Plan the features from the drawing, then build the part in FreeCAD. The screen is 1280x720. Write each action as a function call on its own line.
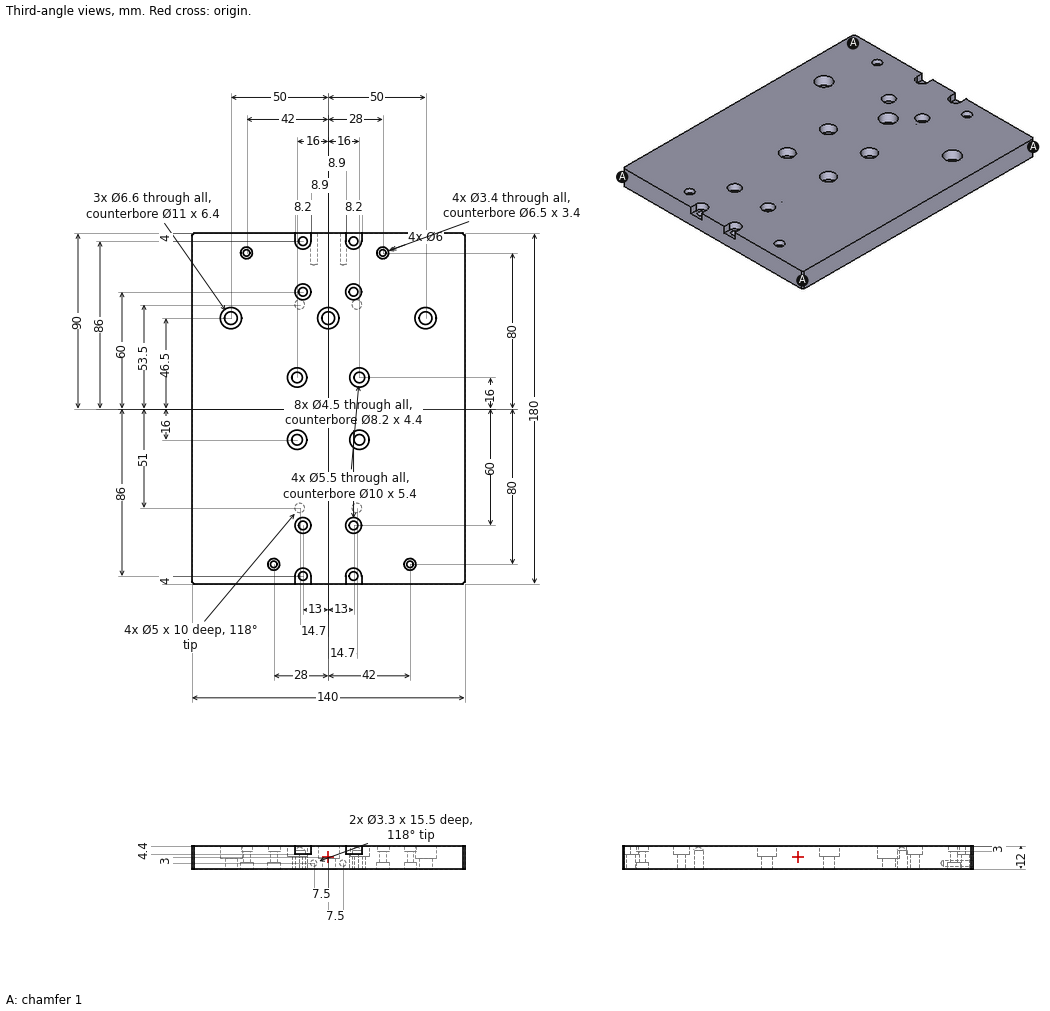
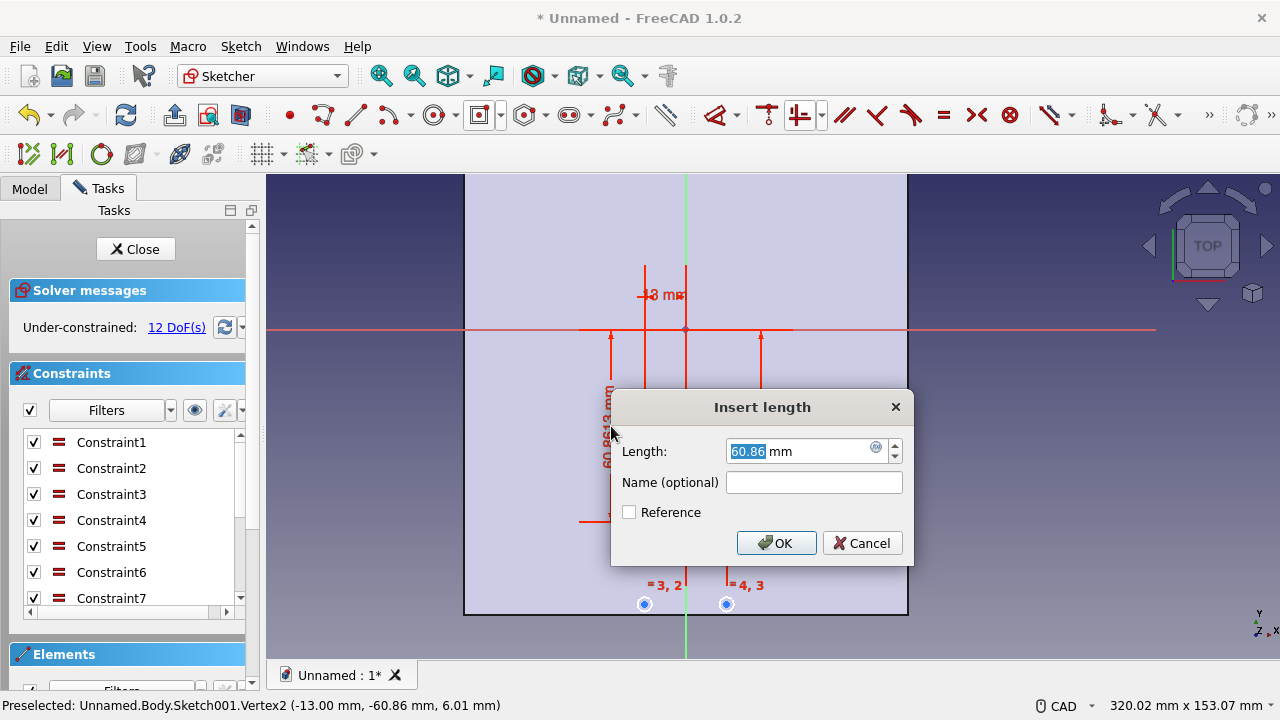
text(60)
key(Return)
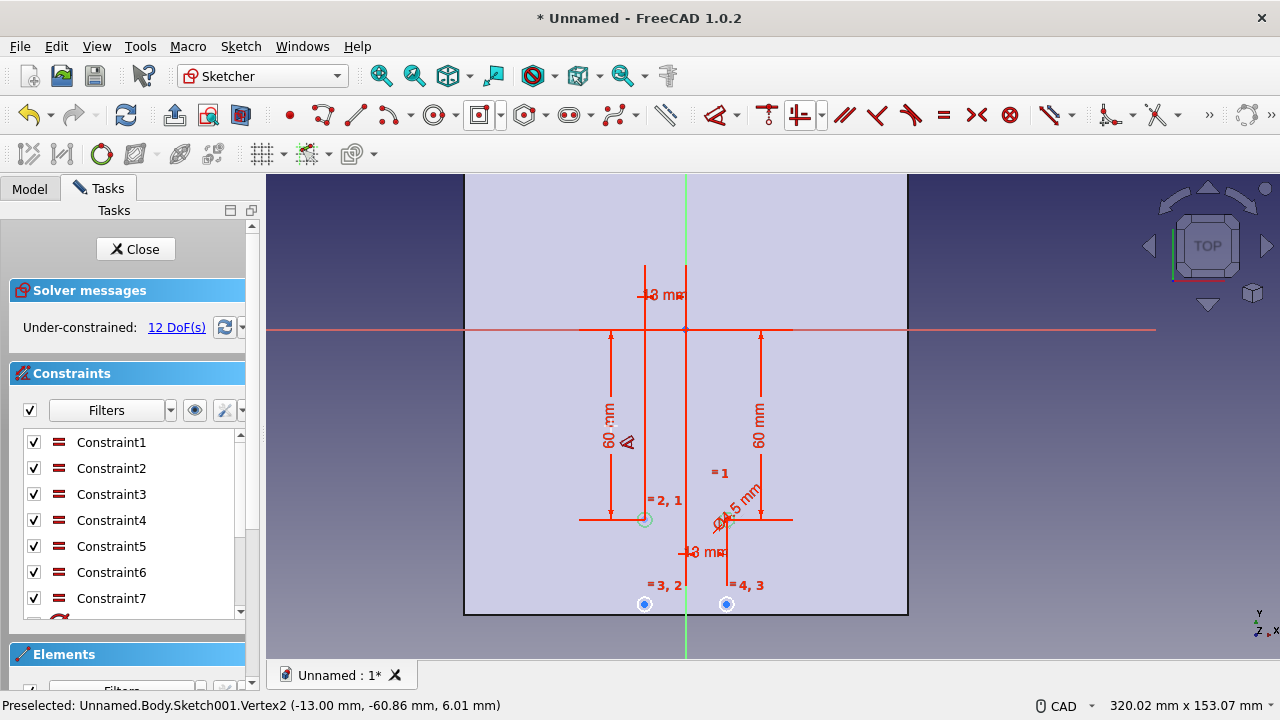
click(645, 604)
click(665, 272)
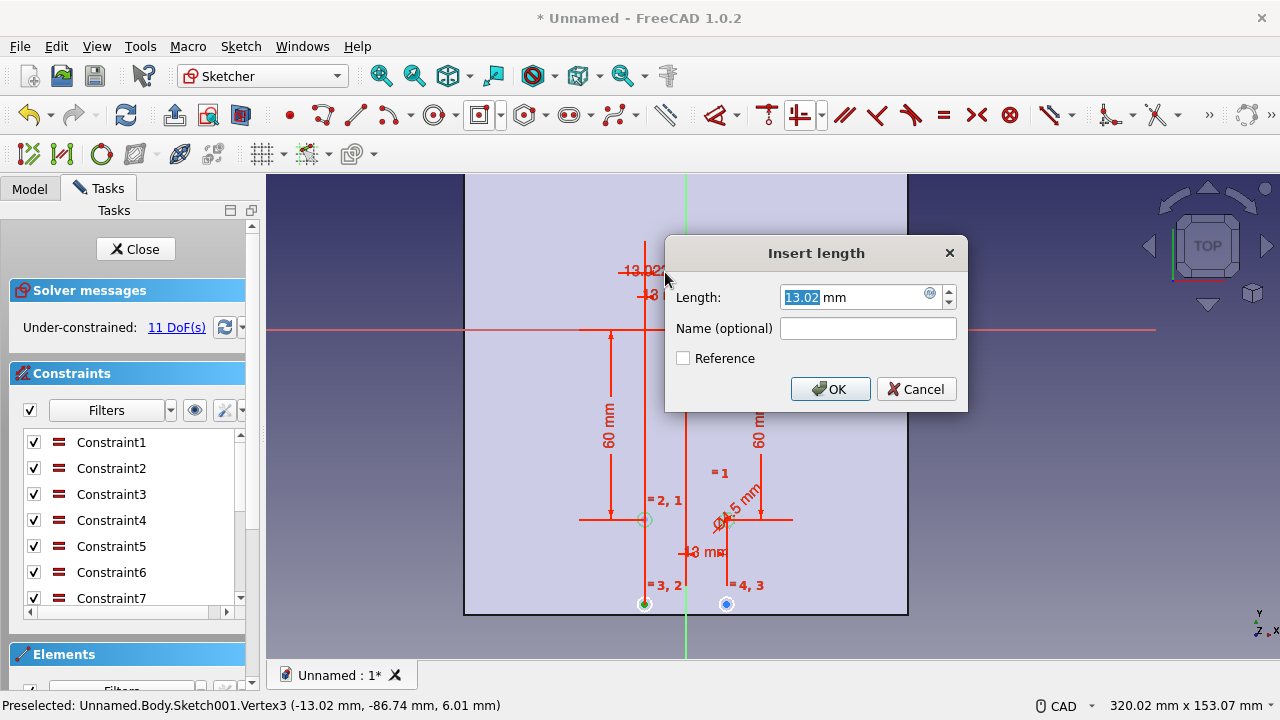
text(13)
key(Return)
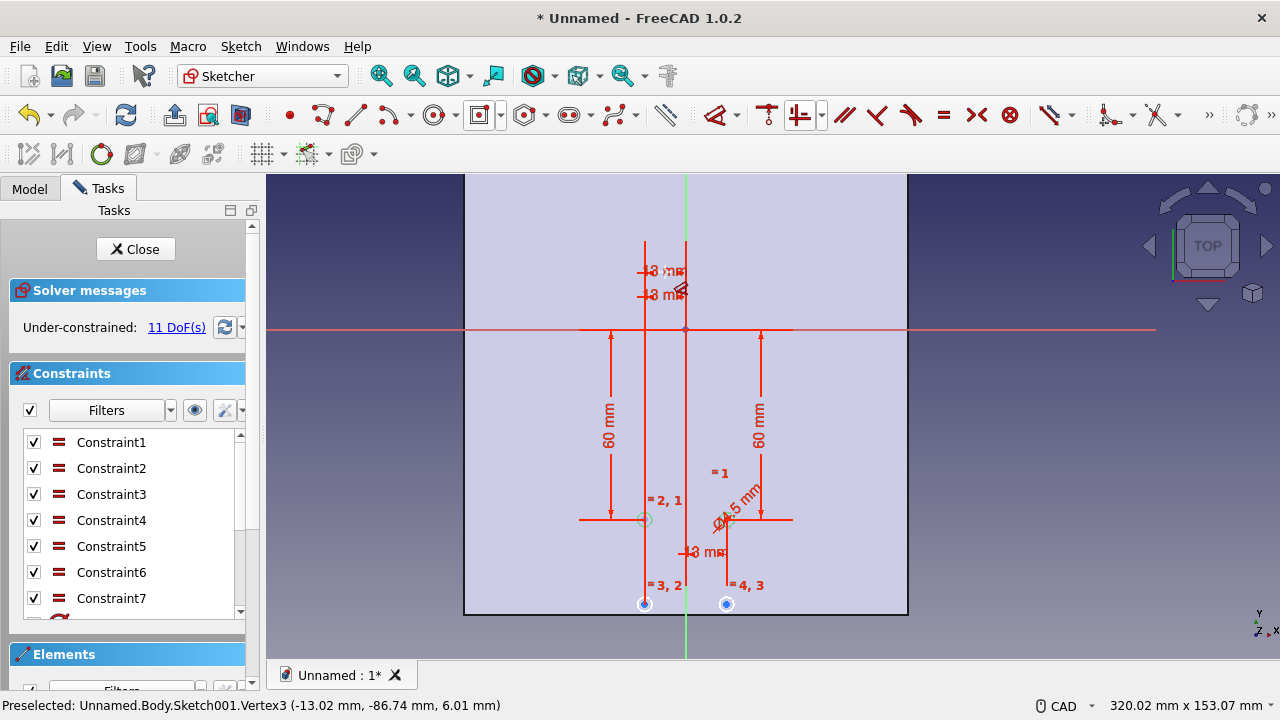
click(645, 604)
click(611, 467)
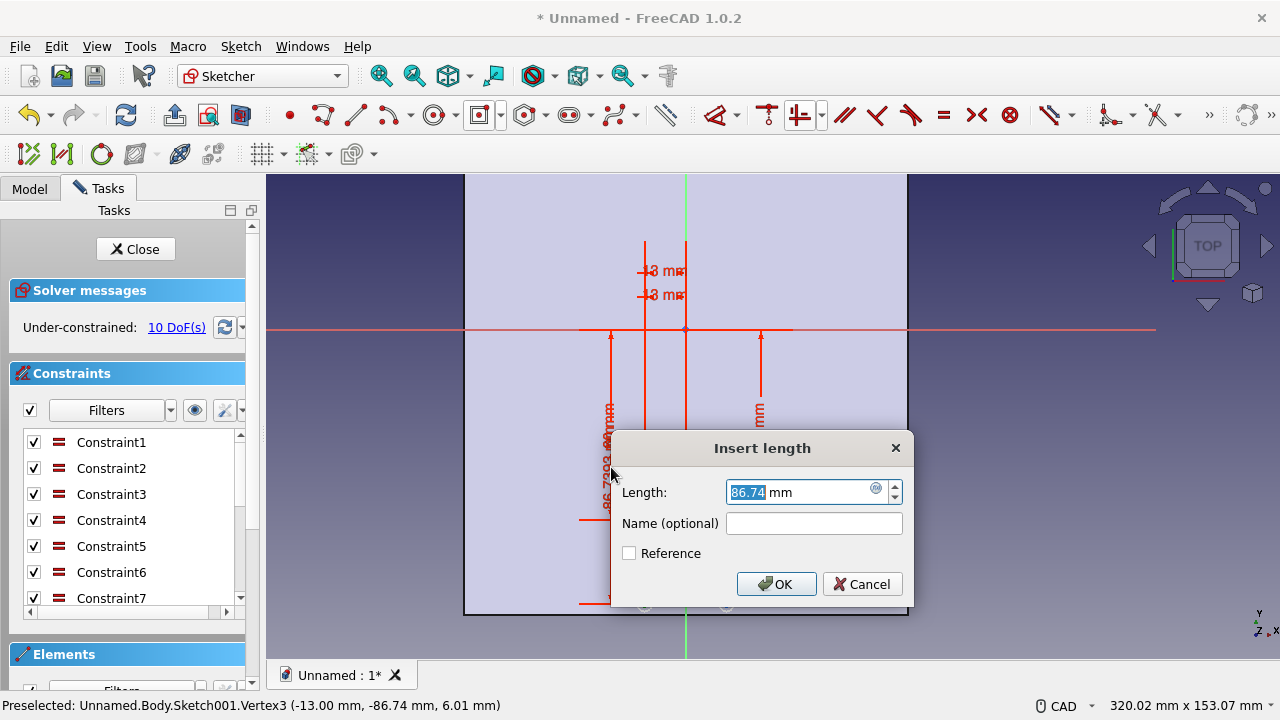
text(86)
key(Return)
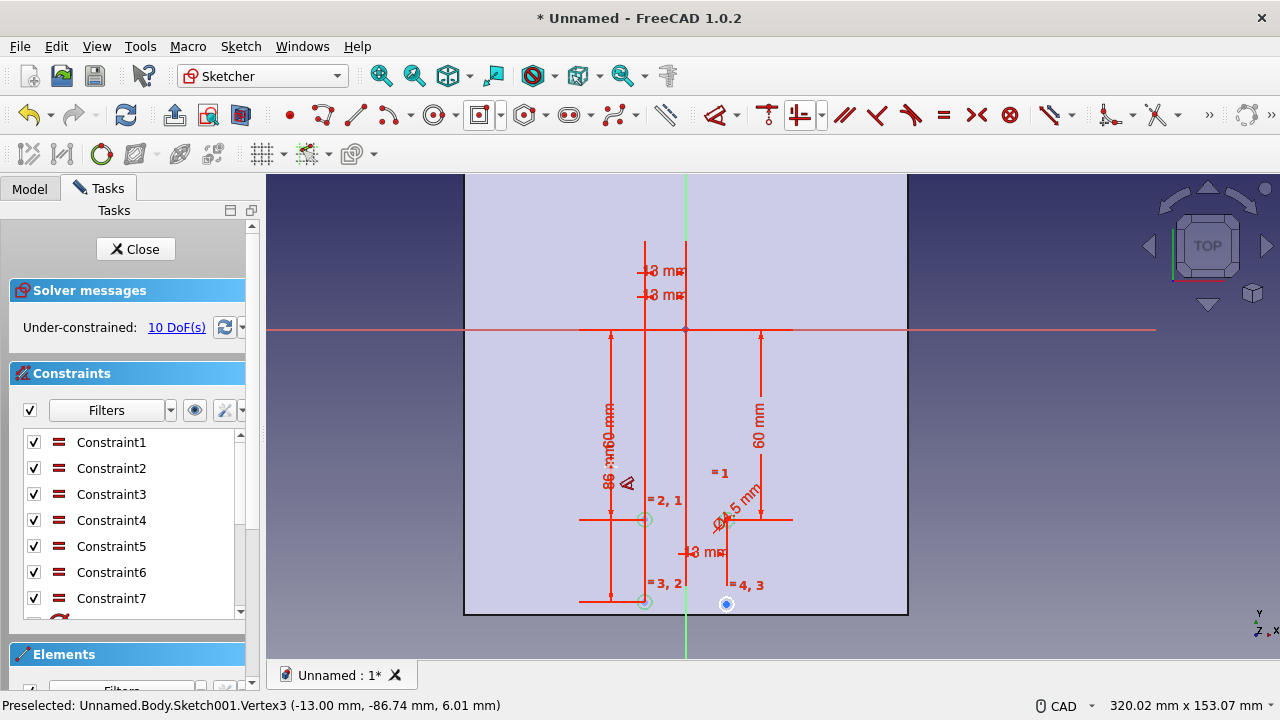
click(727, 604)
click(706, 248)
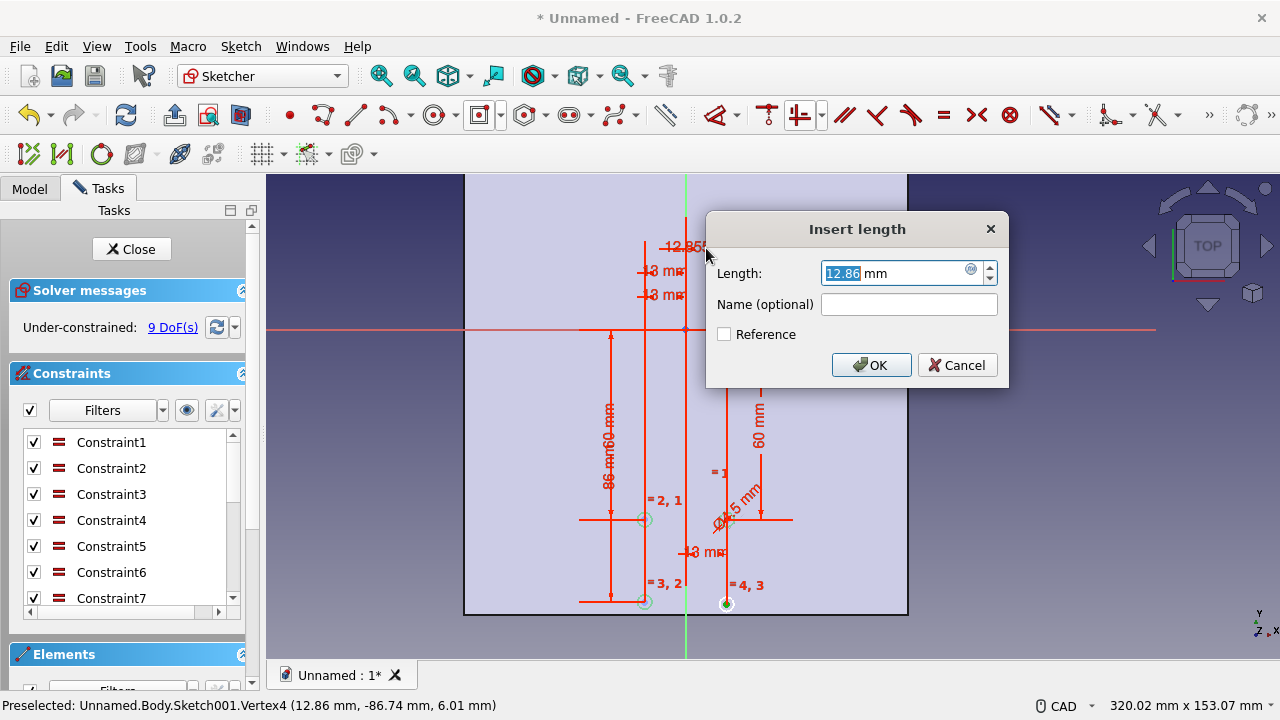
text(13)
key(Return)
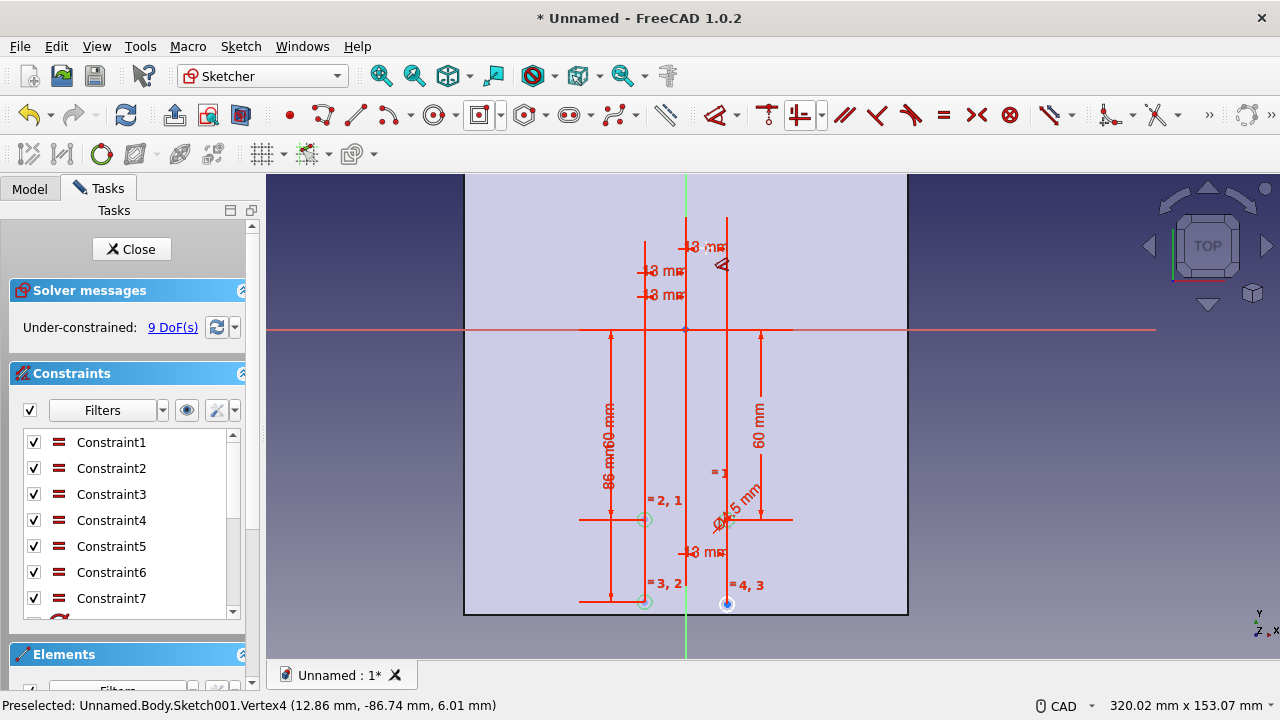
click(727, 604)
click(761, 467)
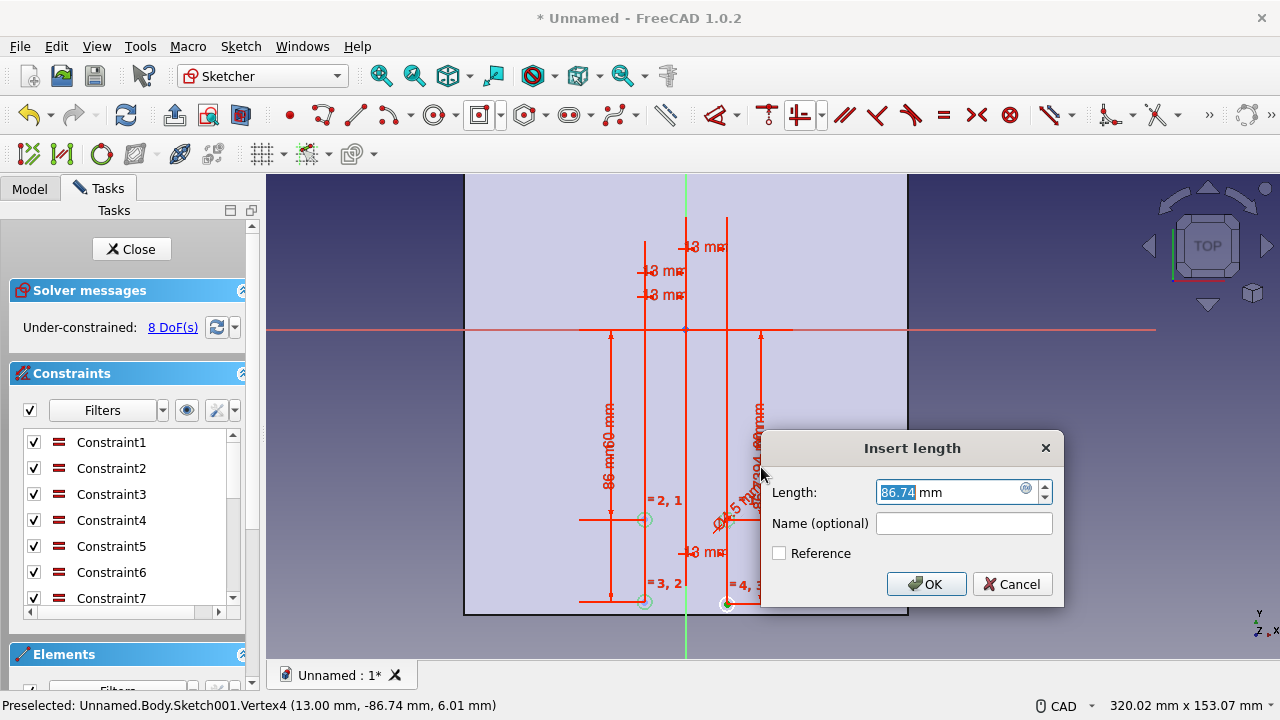
text(86)
key(Return)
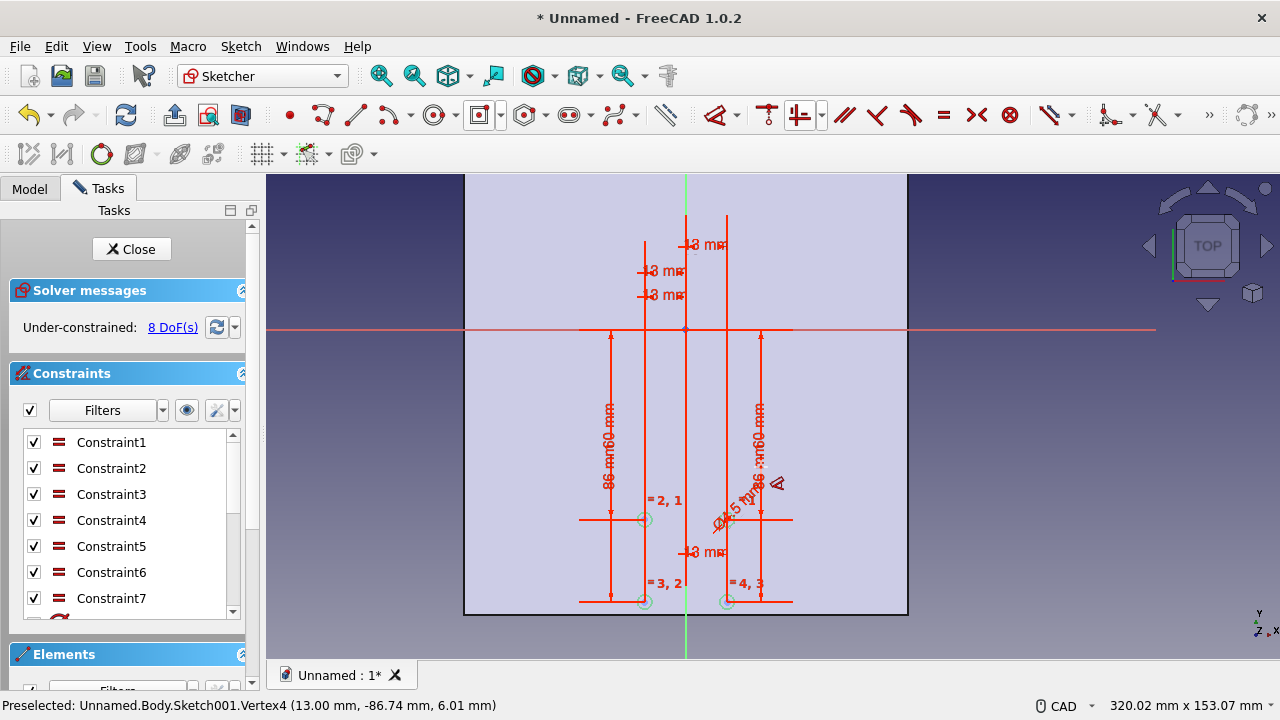
scroll(727, 522, down, 3)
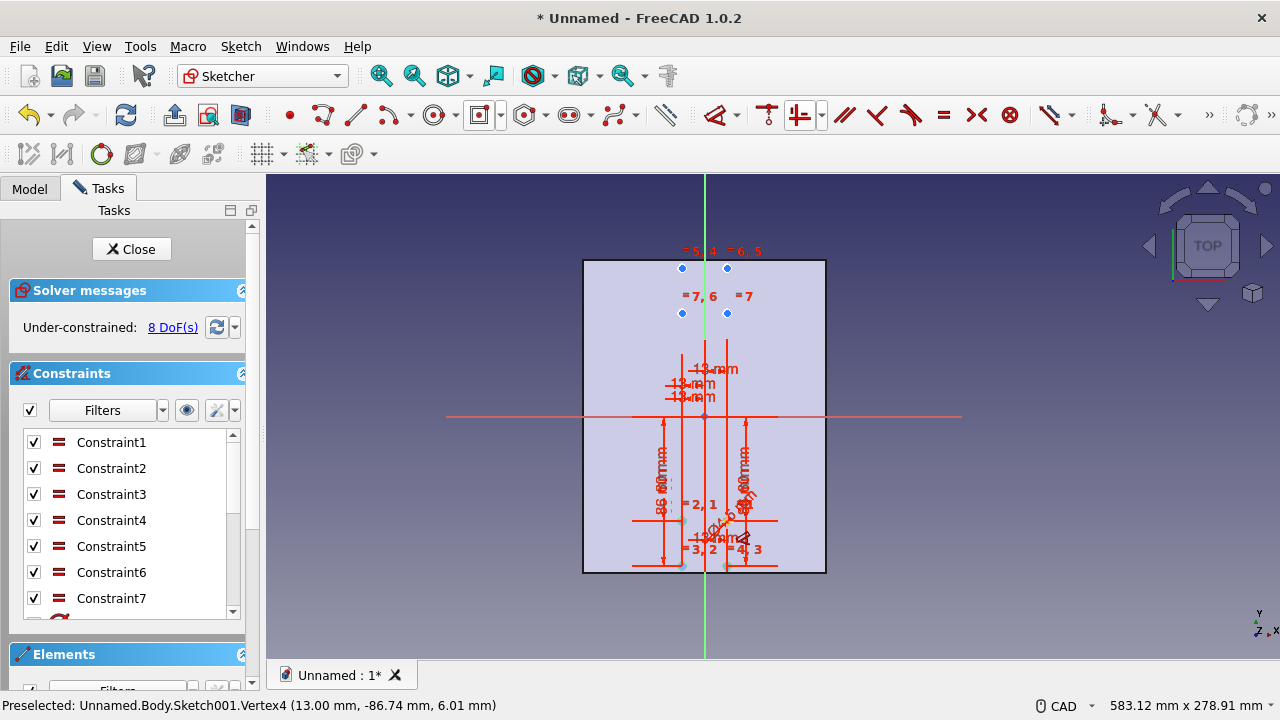
scroll(682, 268, up, 3)